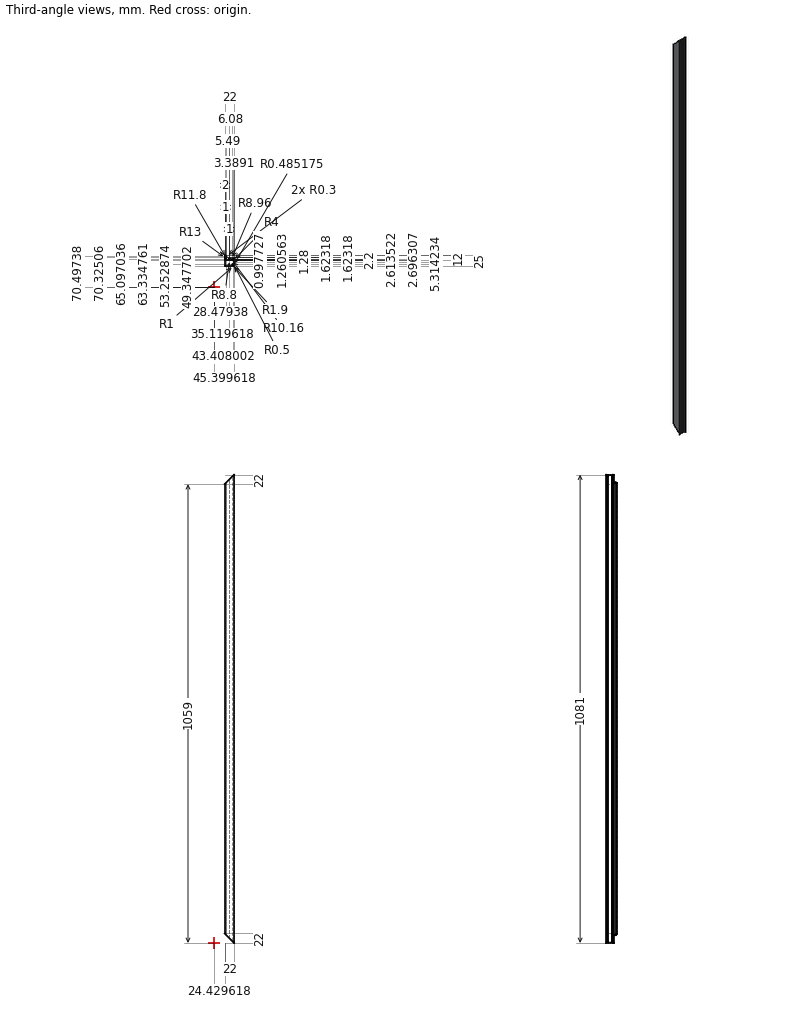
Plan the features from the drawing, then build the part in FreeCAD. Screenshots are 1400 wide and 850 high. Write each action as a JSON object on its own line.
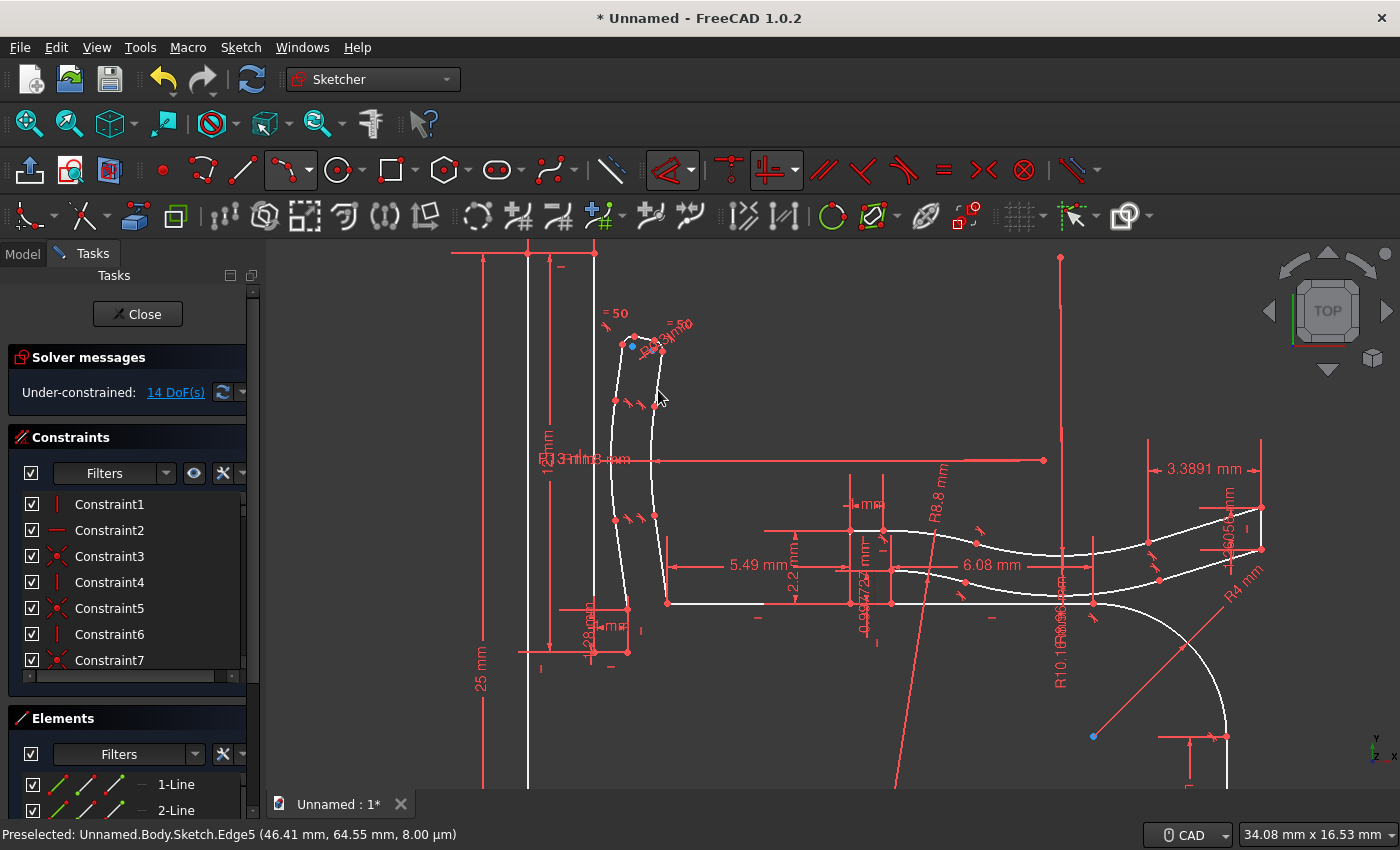
{"action": "left_click", "coordinate": [657, 390]}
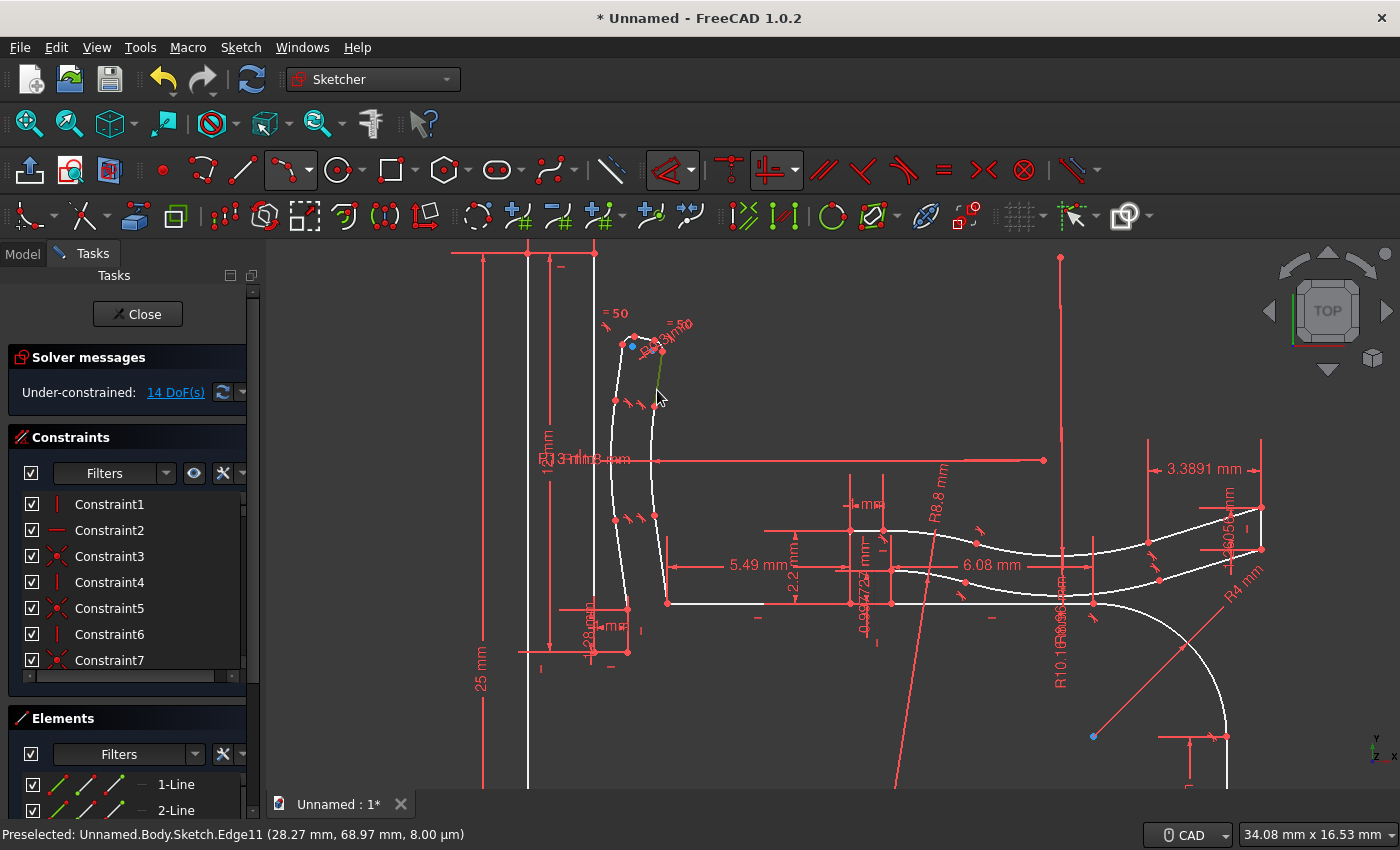
{"action": "key", "text": "i"}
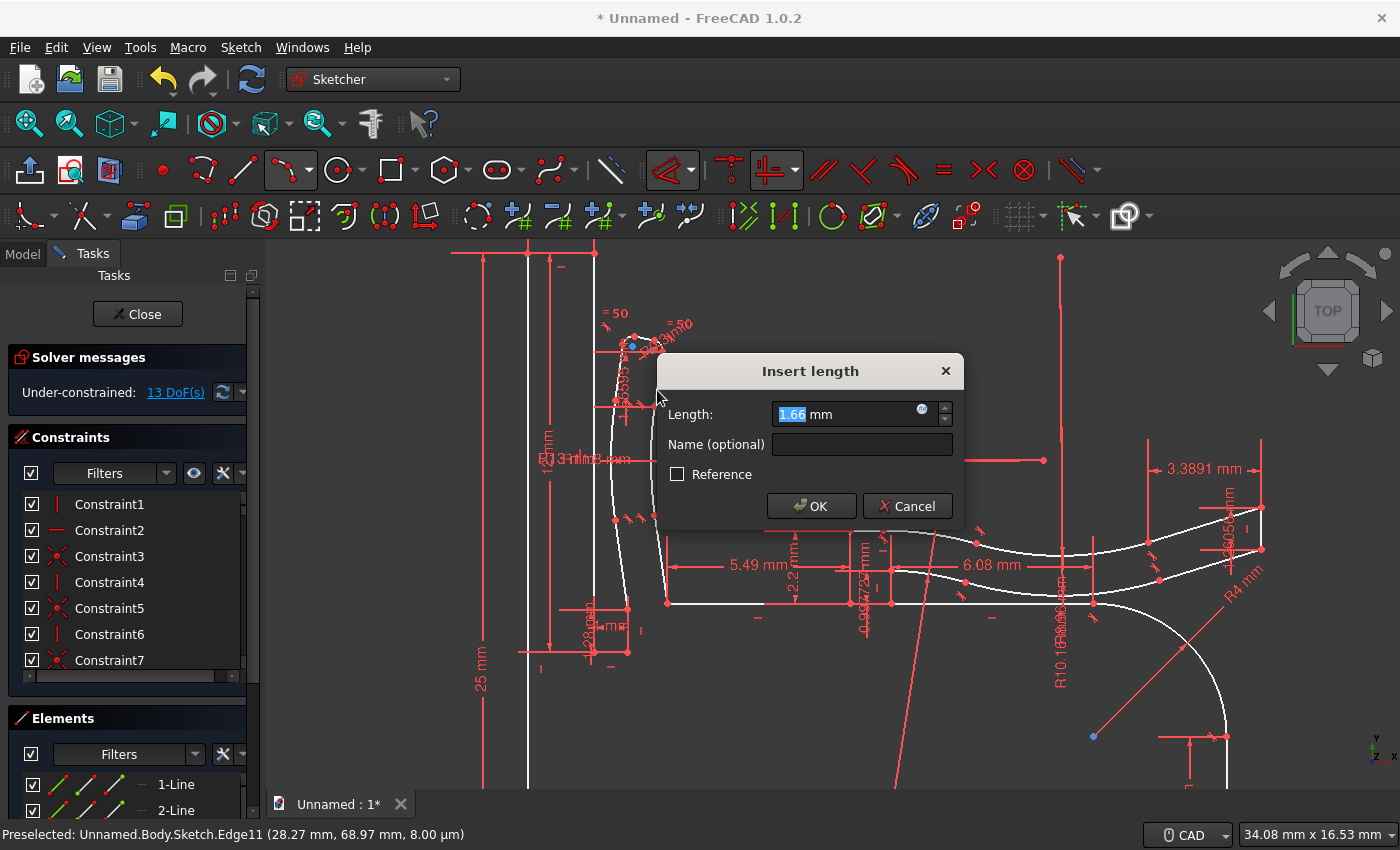
{"action": "type", "text": "1.62318"}
{"action": "key", "text": "Return"}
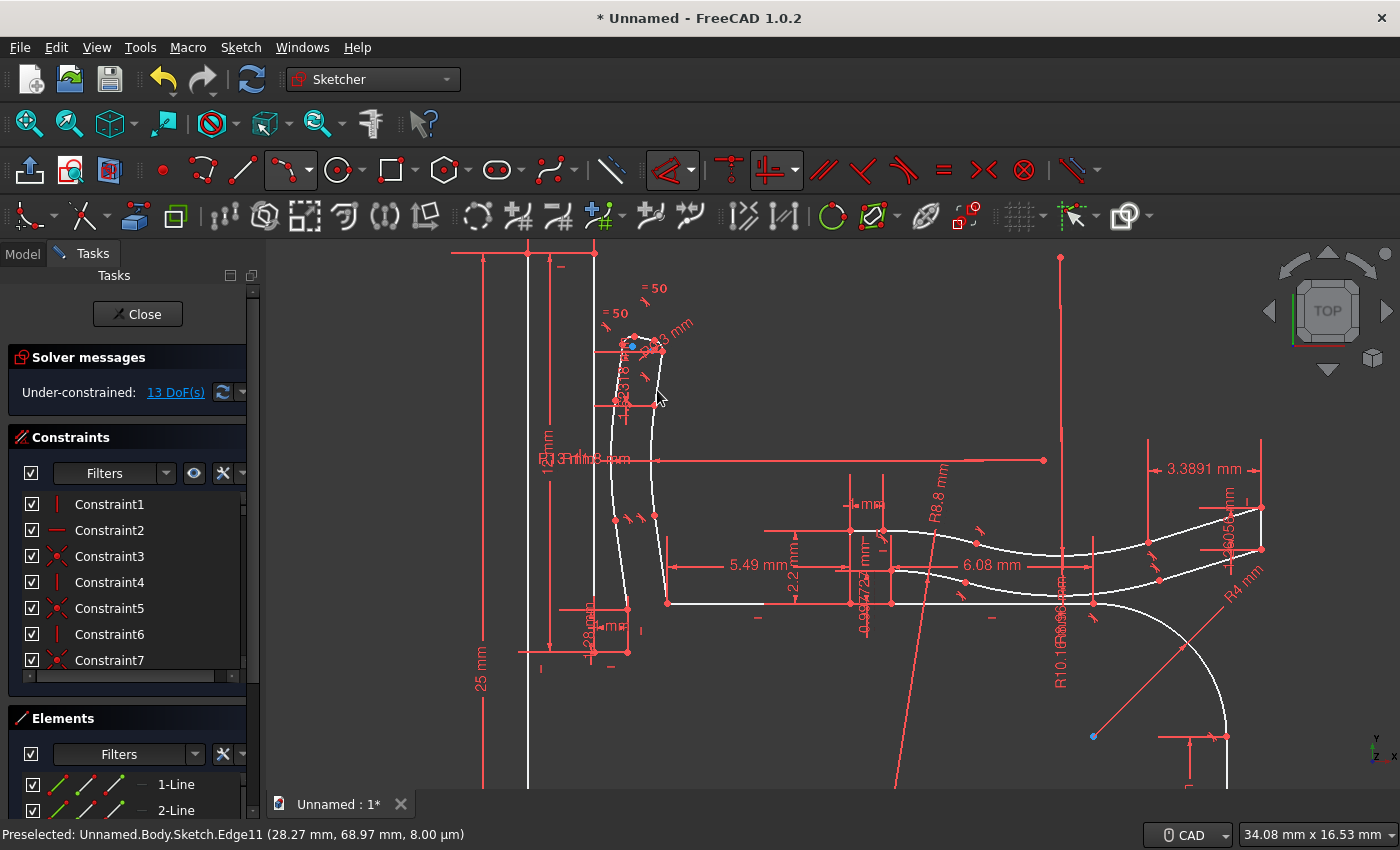
{"action": "left_click", "coordinate": [617, 390]}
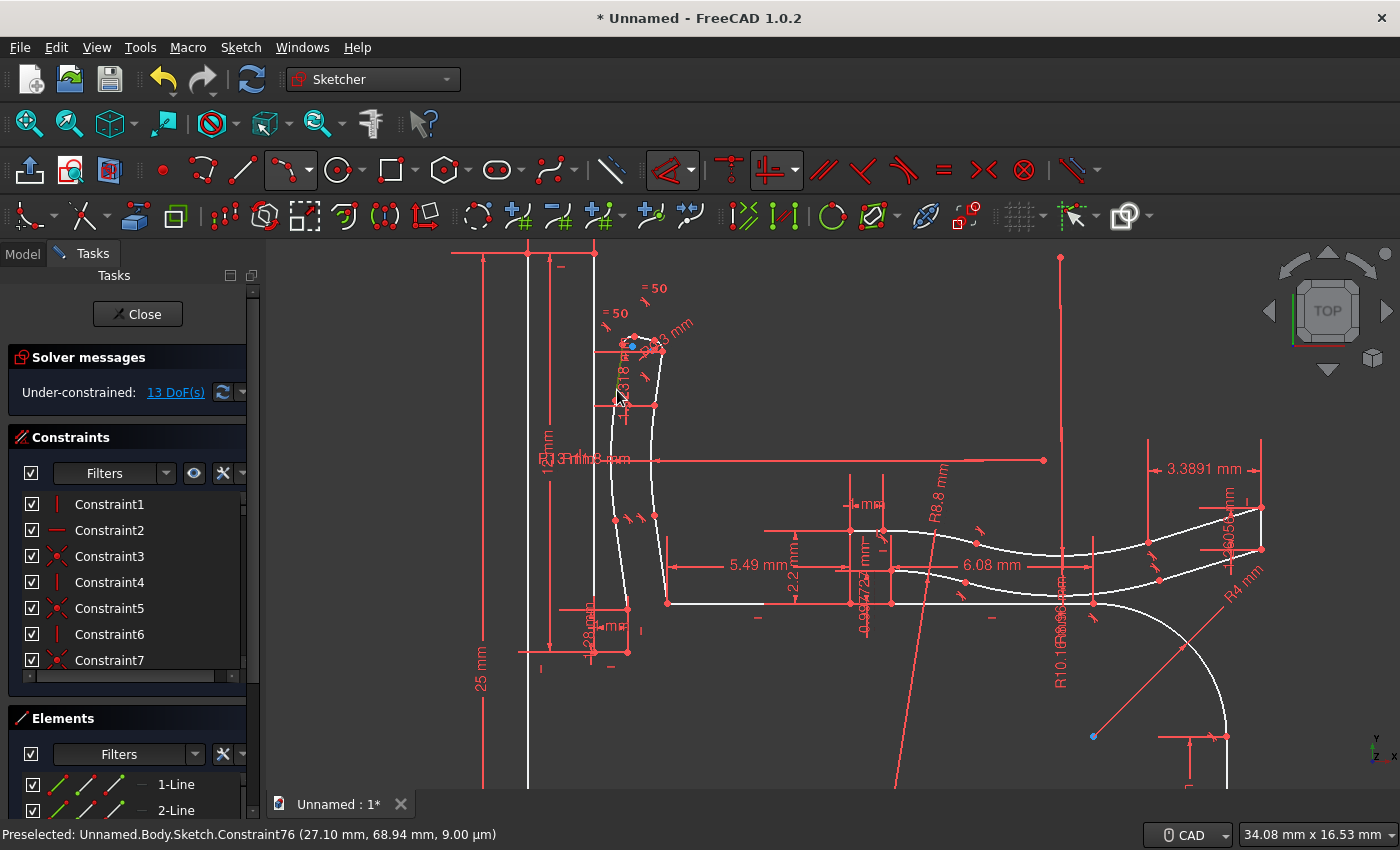
{"action": "key", "text": "i"}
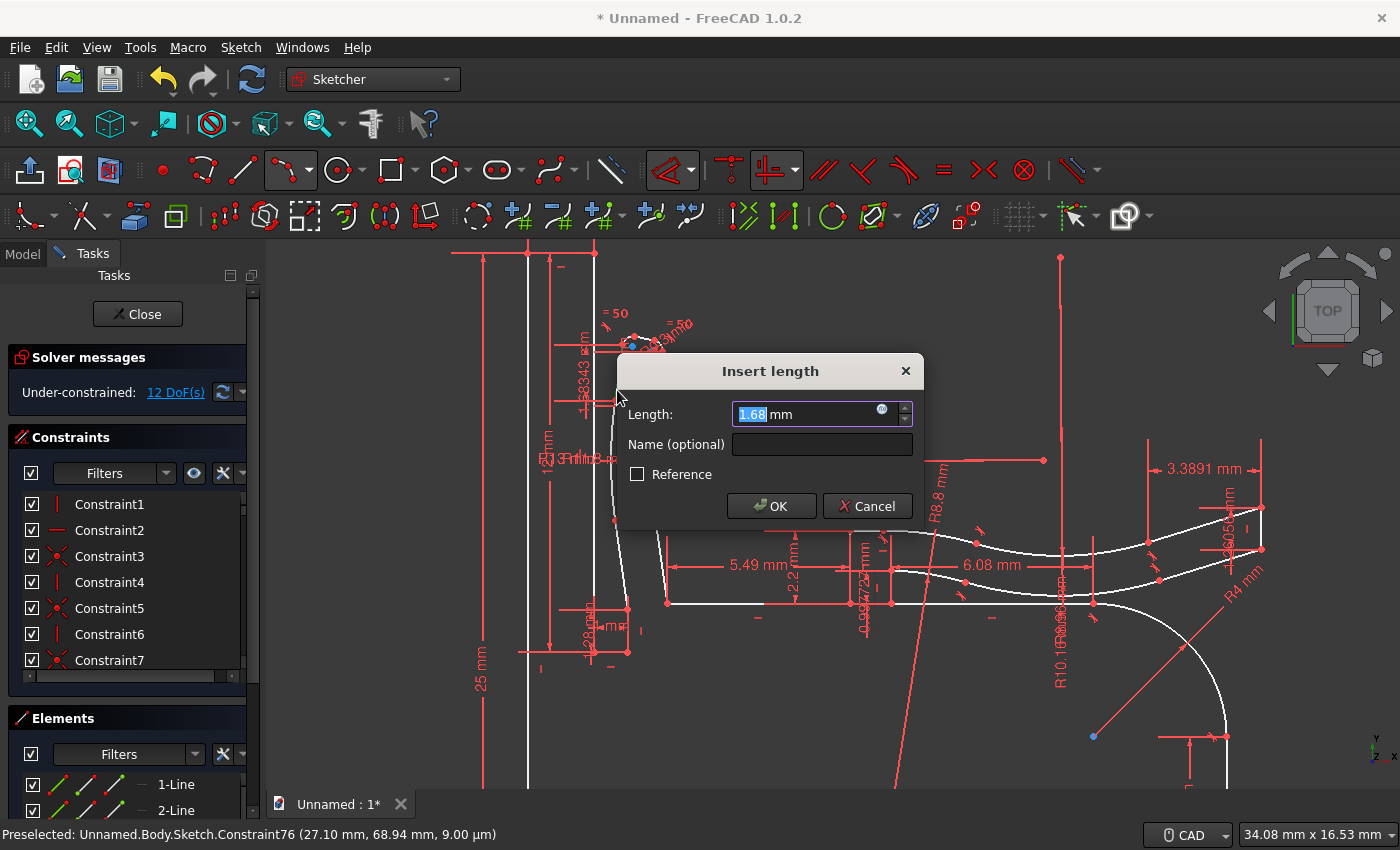
{"action": "type", "text": "1.62318"}
{"action": "key", "text": "Return"}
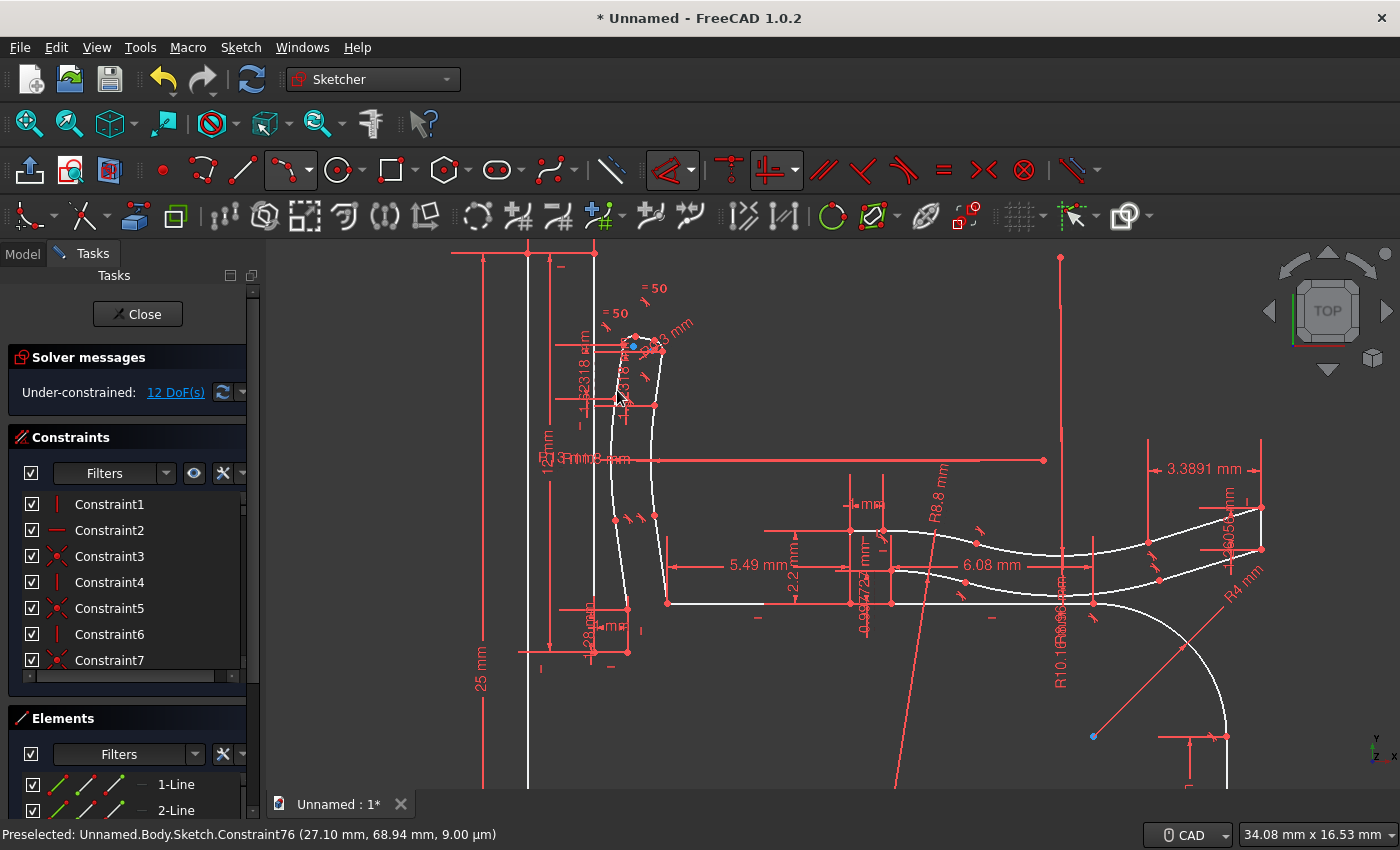
{"action": "scroll", "coordinate": [662, 352], "scroll_direction": "up", "scroll_amount": 2}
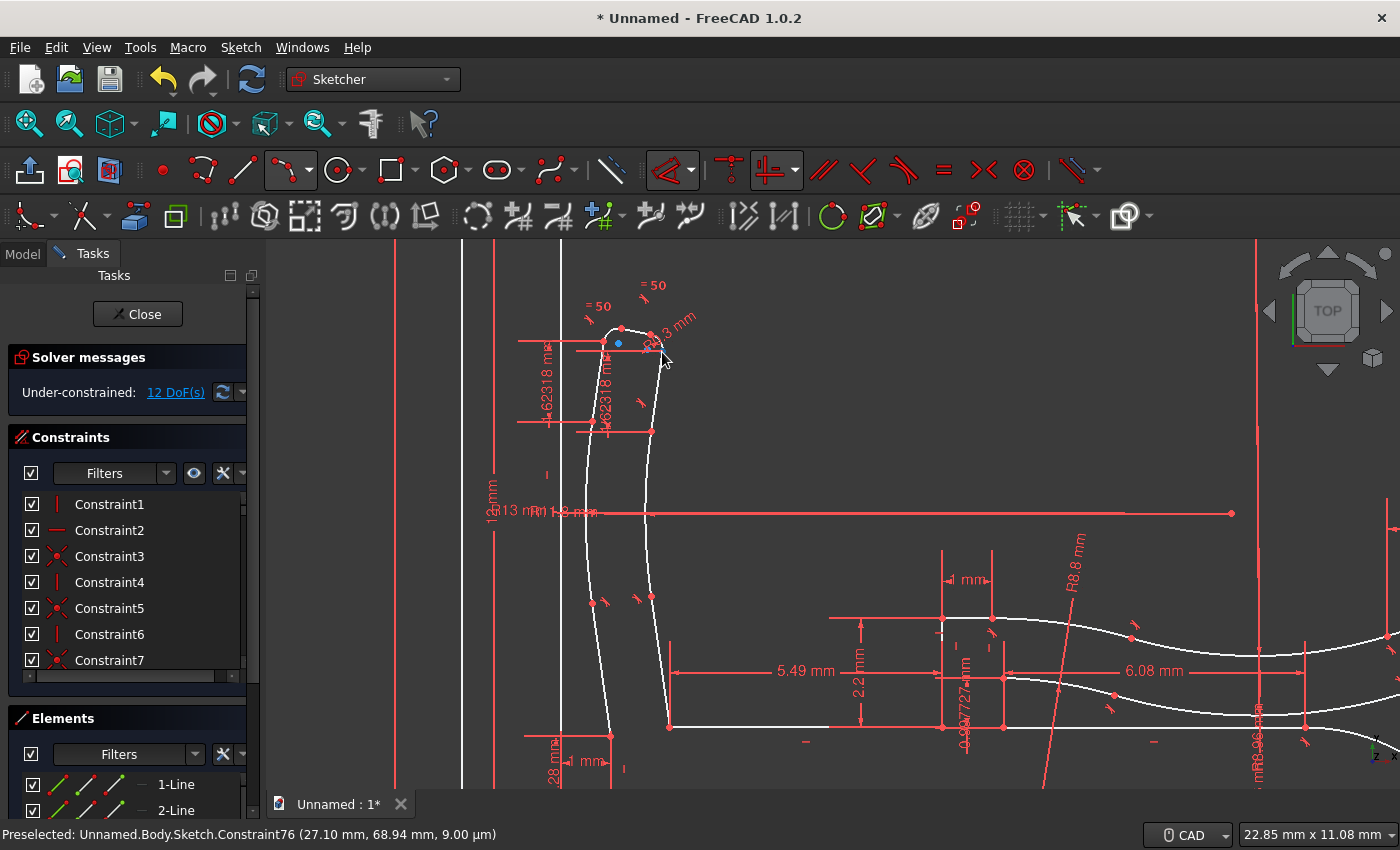
{"action": "left_click", "coordinate": [662, 351]}